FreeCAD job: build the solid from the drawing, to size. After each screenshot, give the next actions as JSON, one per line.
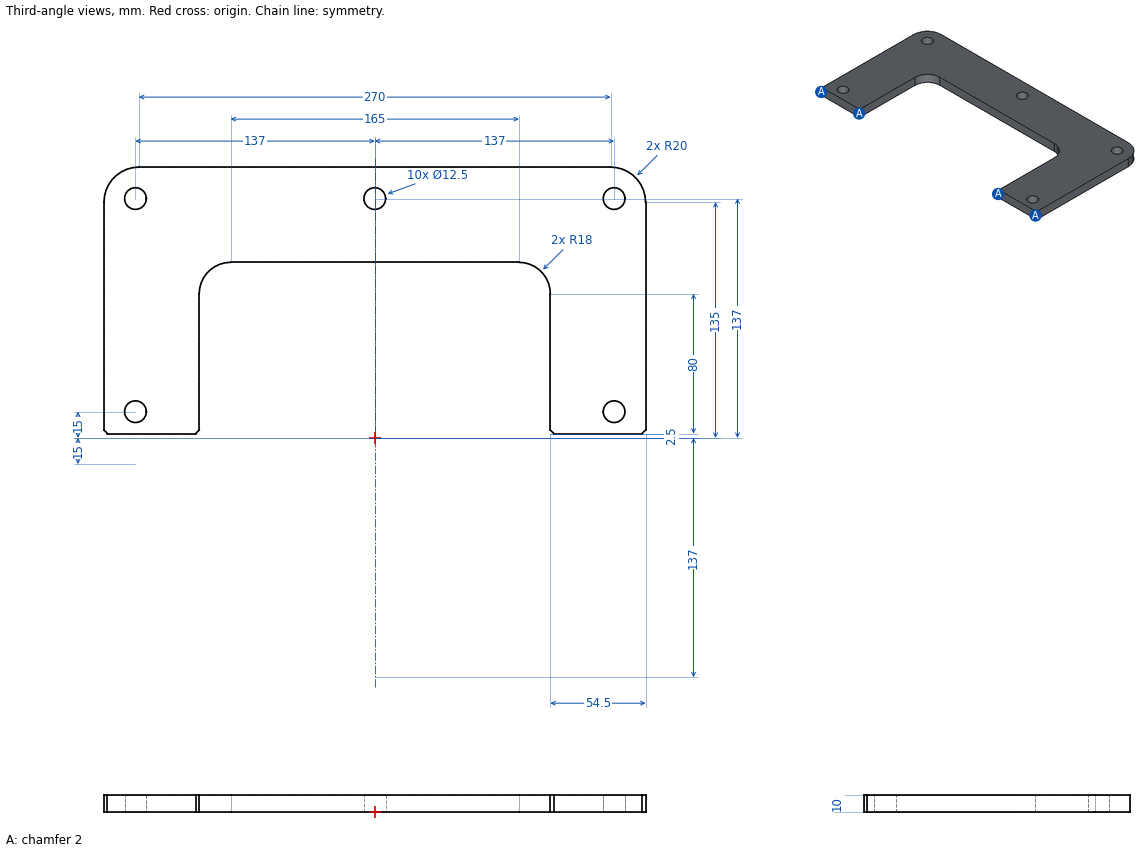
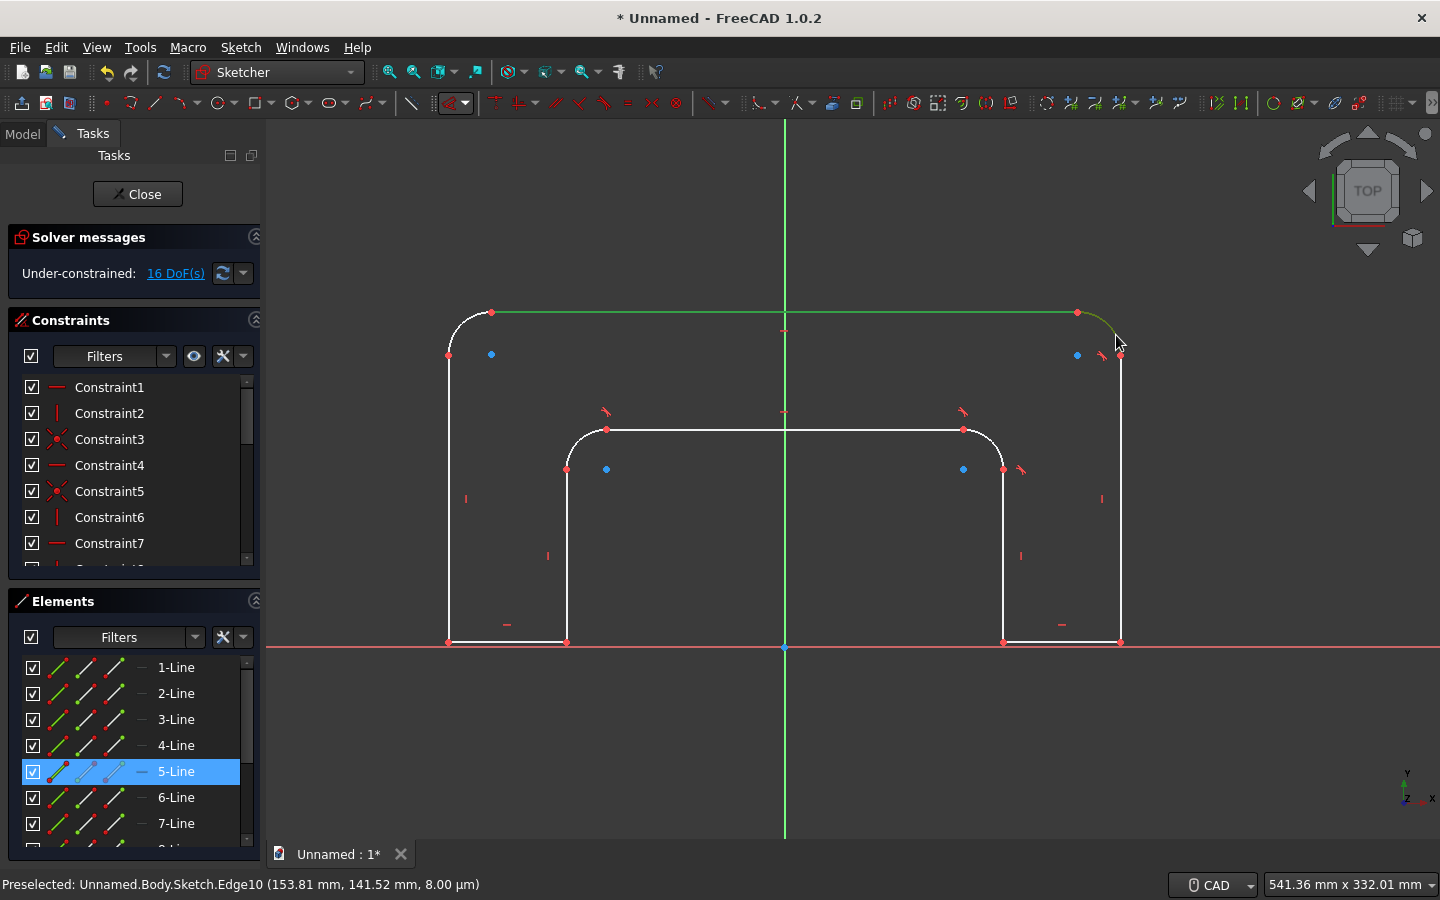
{"action": "key", "text": "t"}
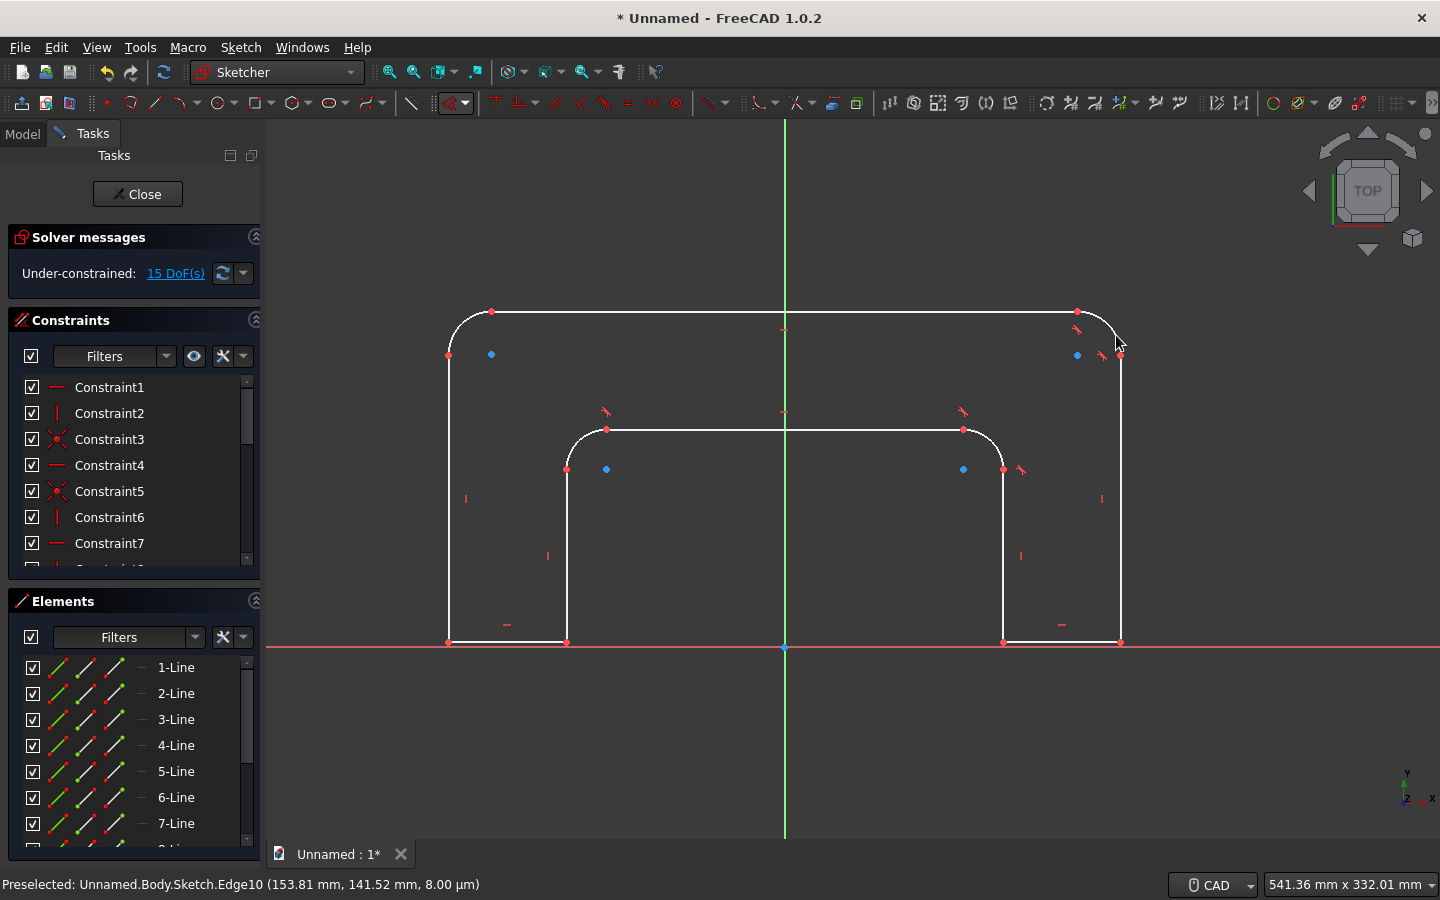
{"action": "left_click", "coordinate": [901, 312]}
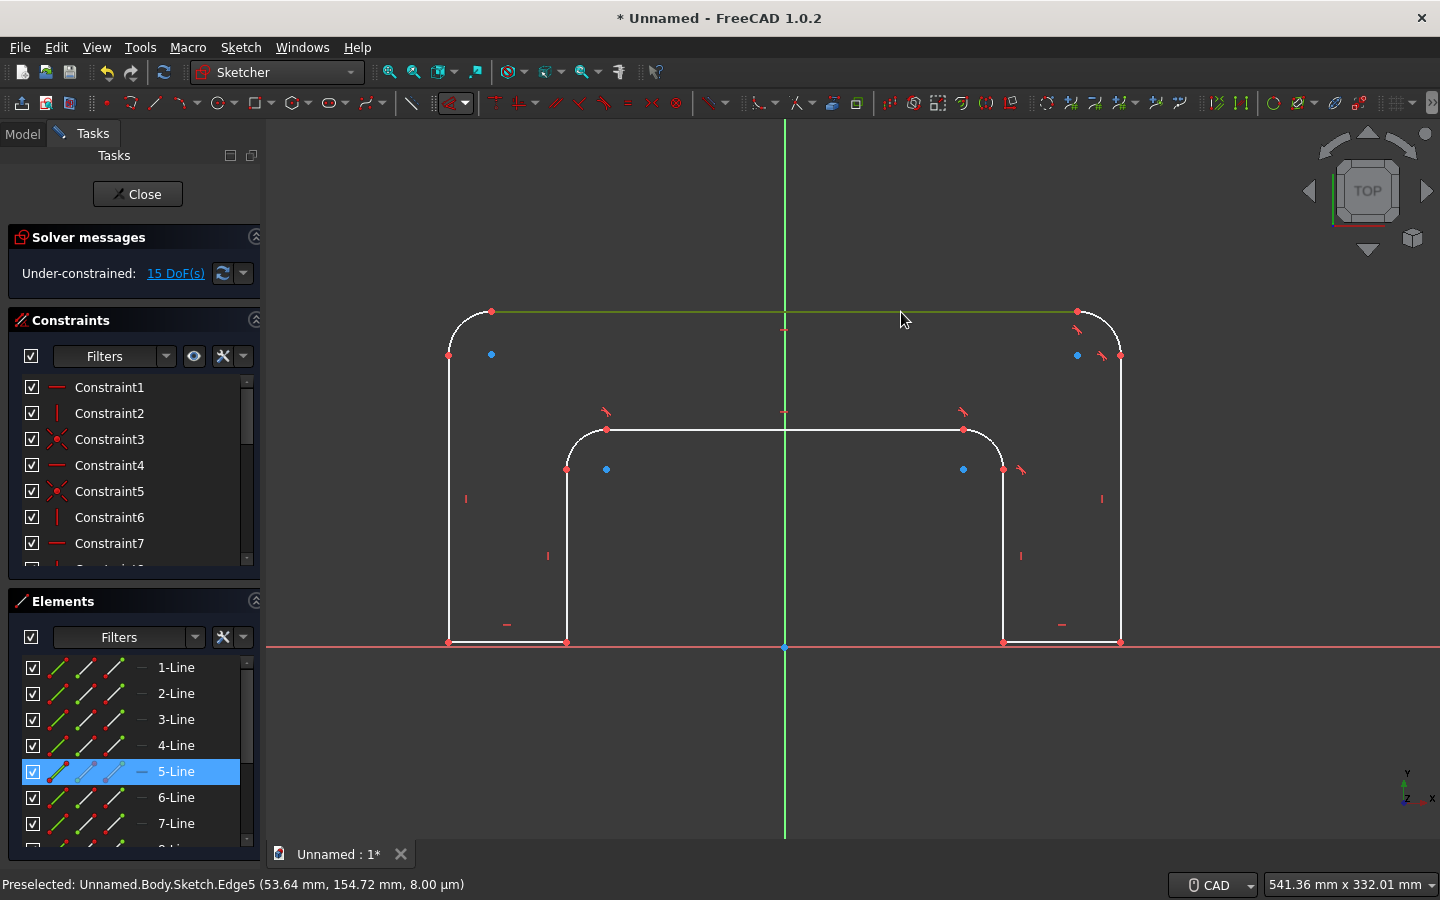
{"action": "left_click", "coordinate": [472, 316]}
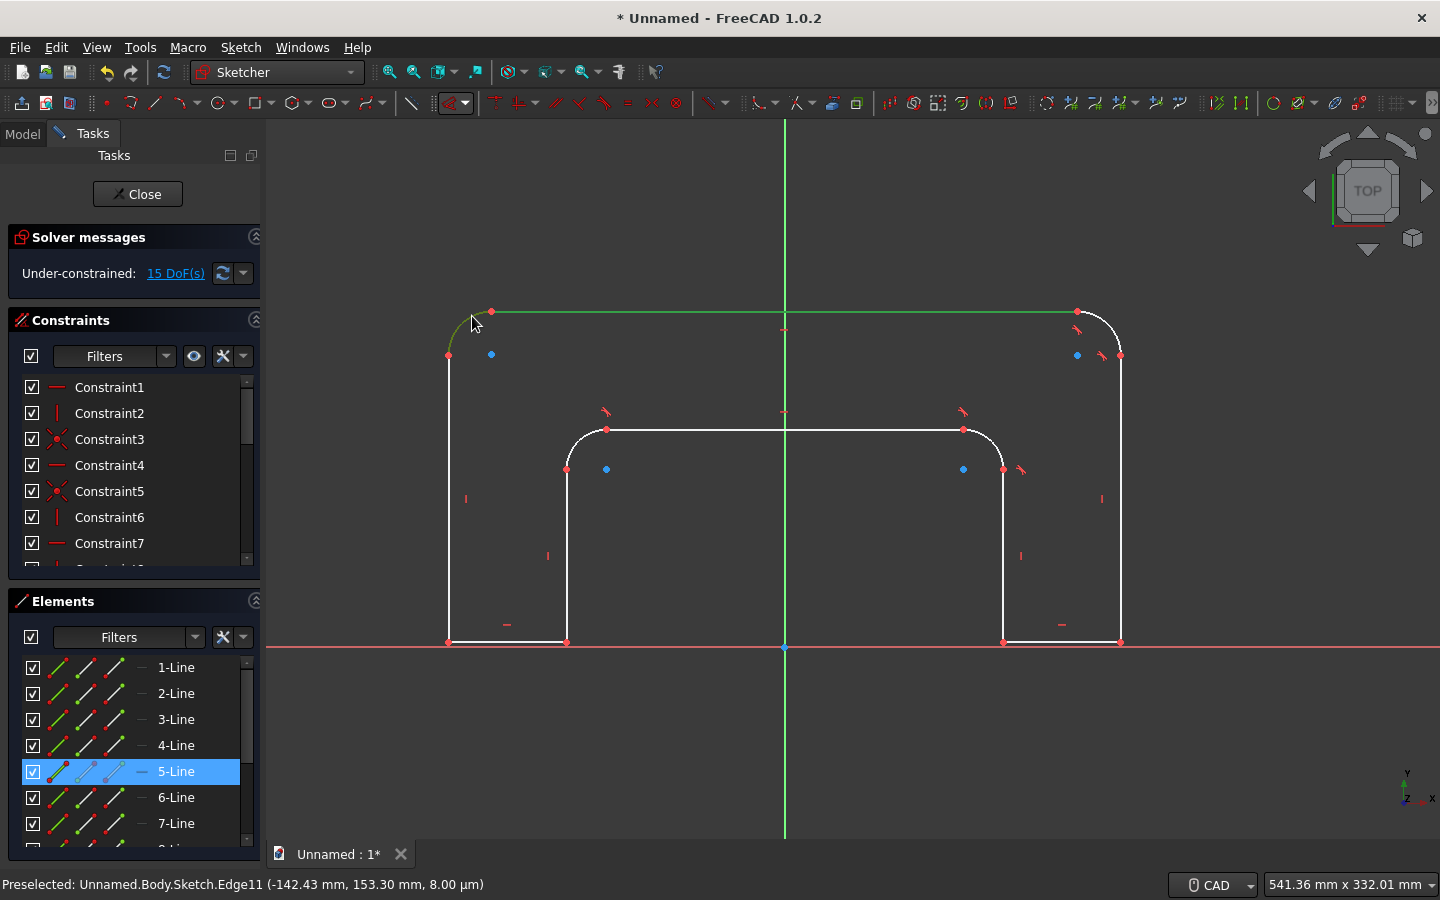
{"action": "left_click", "coordinate": [604, 104]}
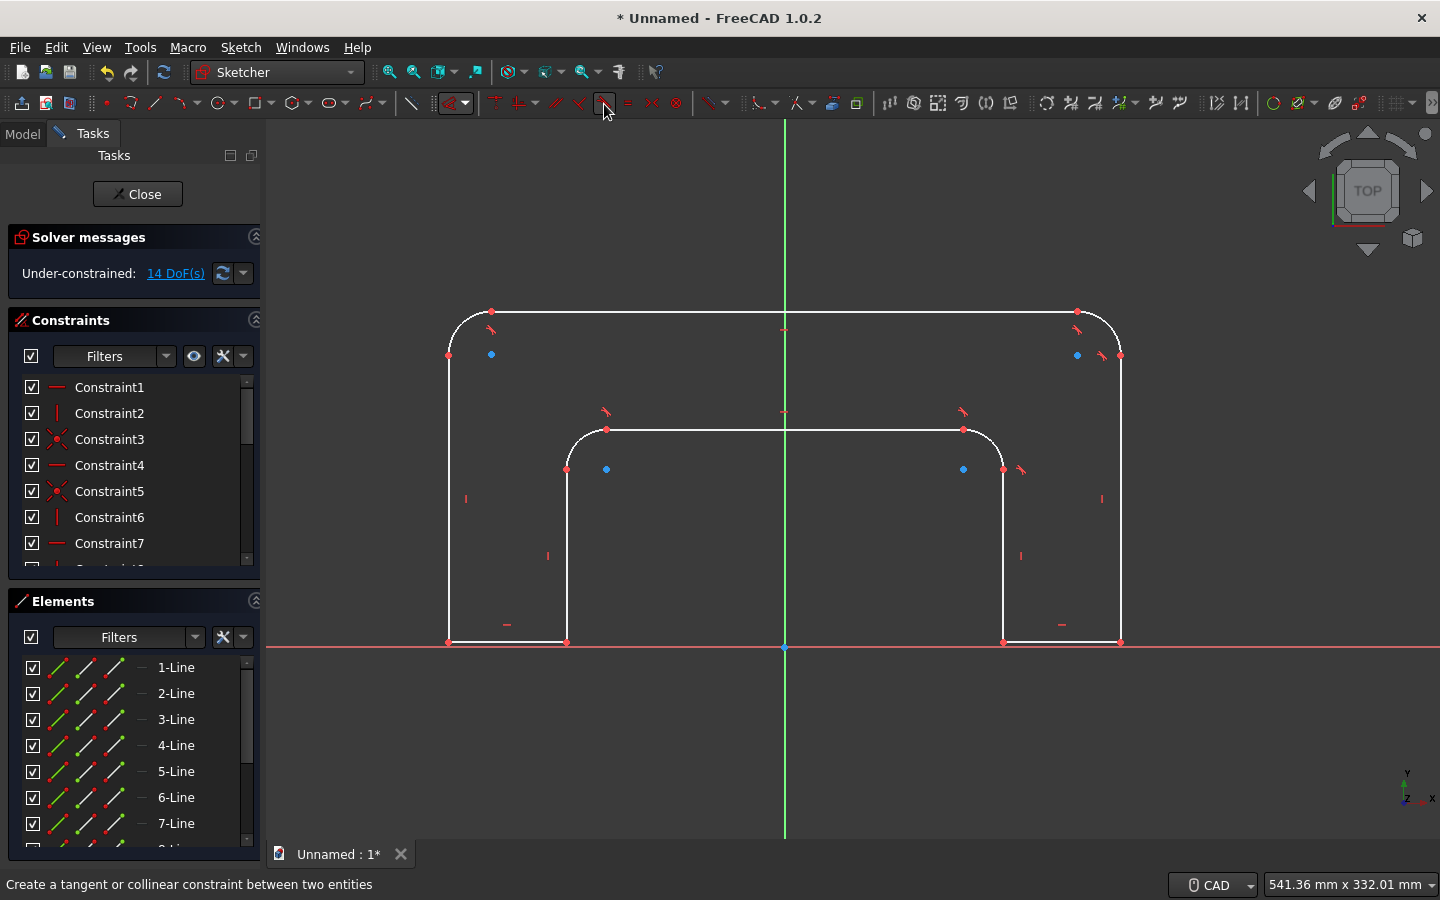
{"action": "left_click", "coordinate": [449, 441]}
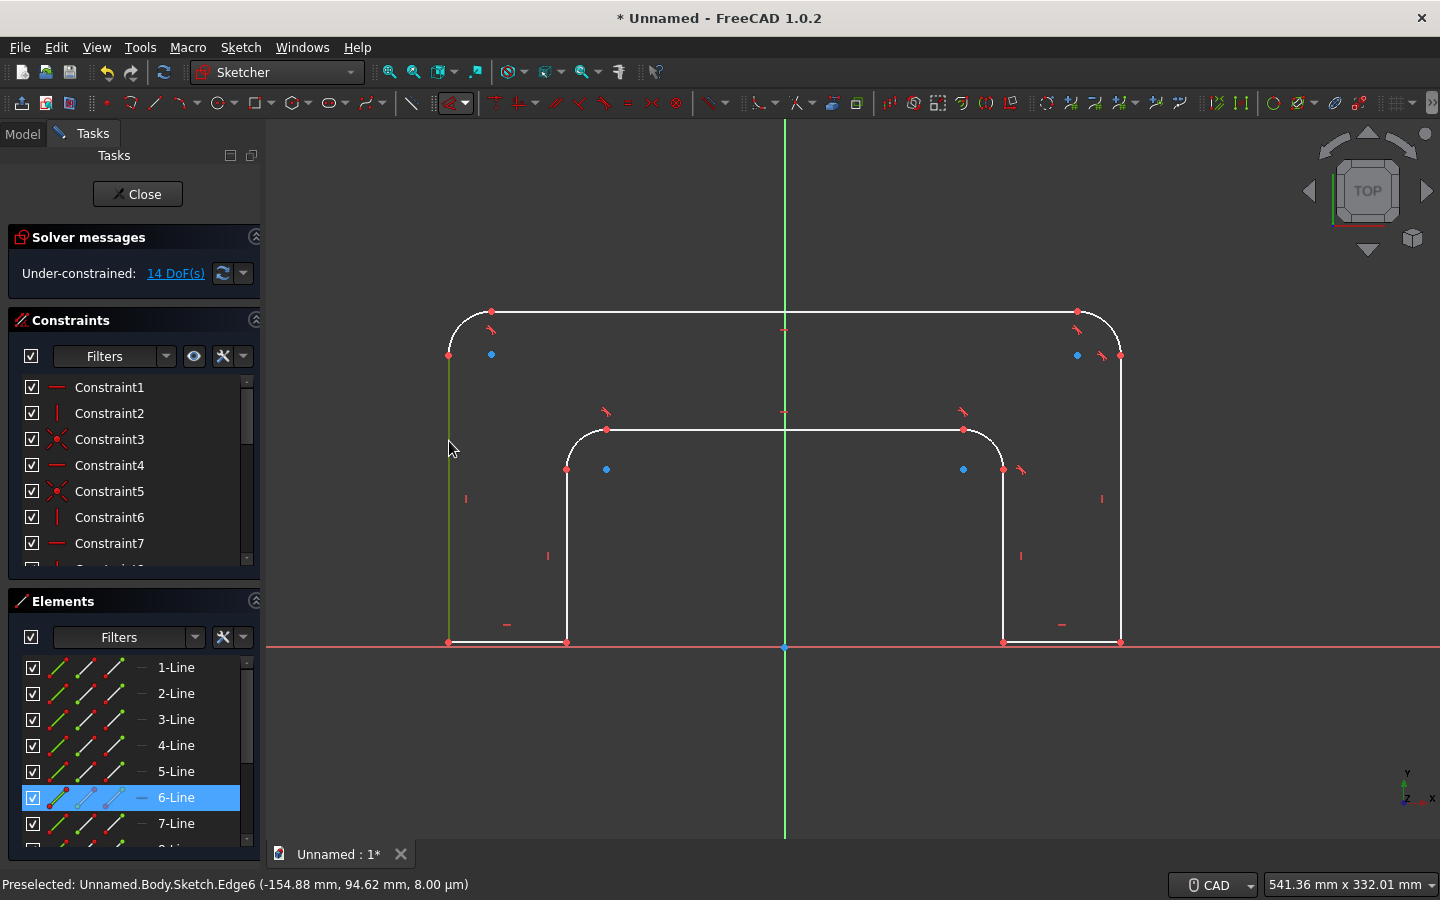
{"action": "left_click", "coordinate": [472, 316]}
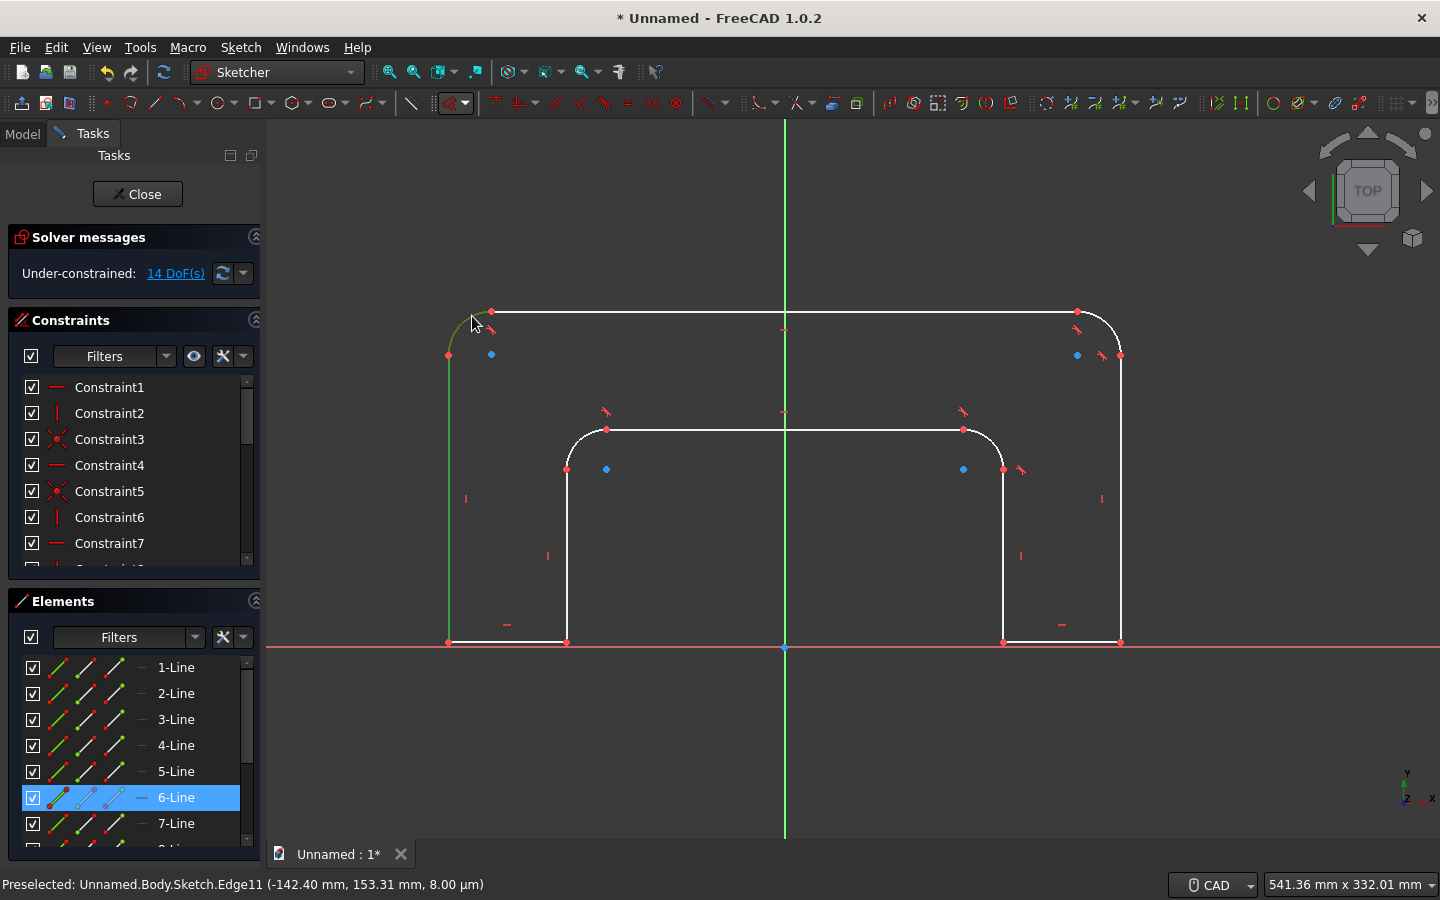
{"action": "key", "text": "t"}